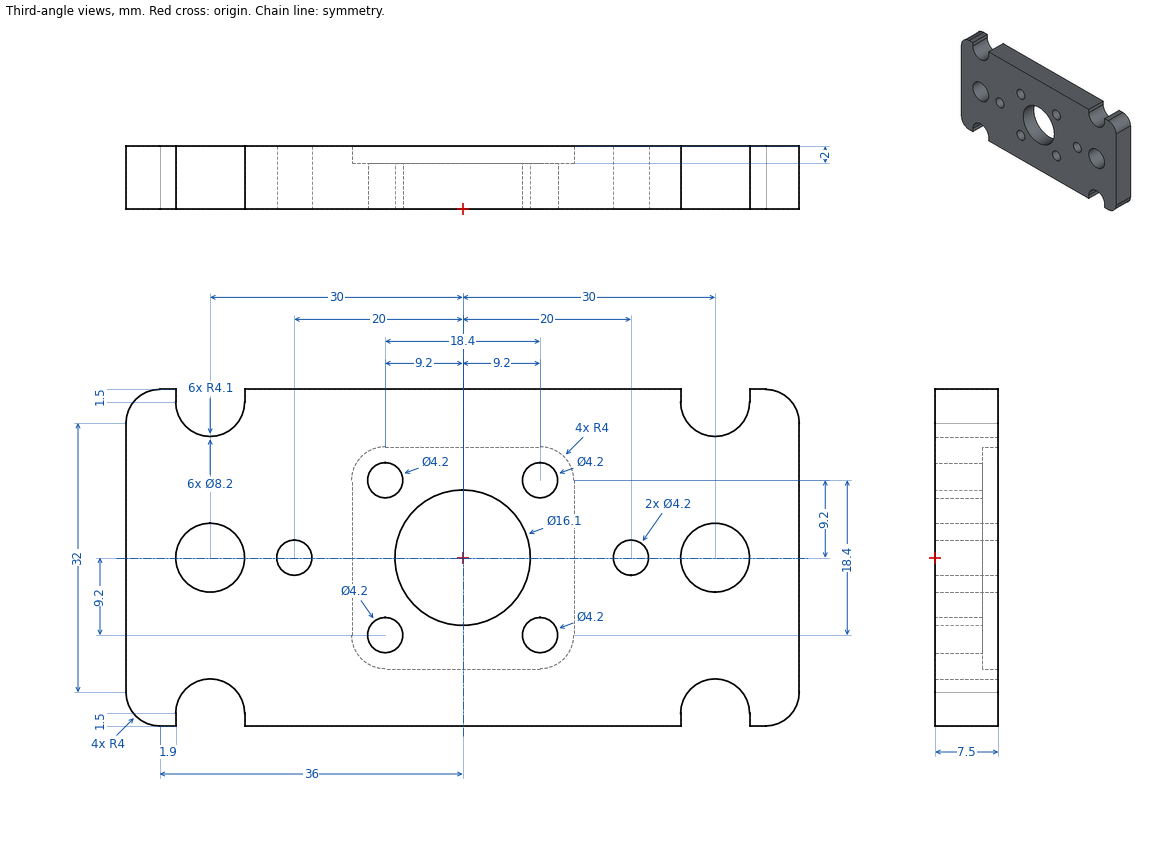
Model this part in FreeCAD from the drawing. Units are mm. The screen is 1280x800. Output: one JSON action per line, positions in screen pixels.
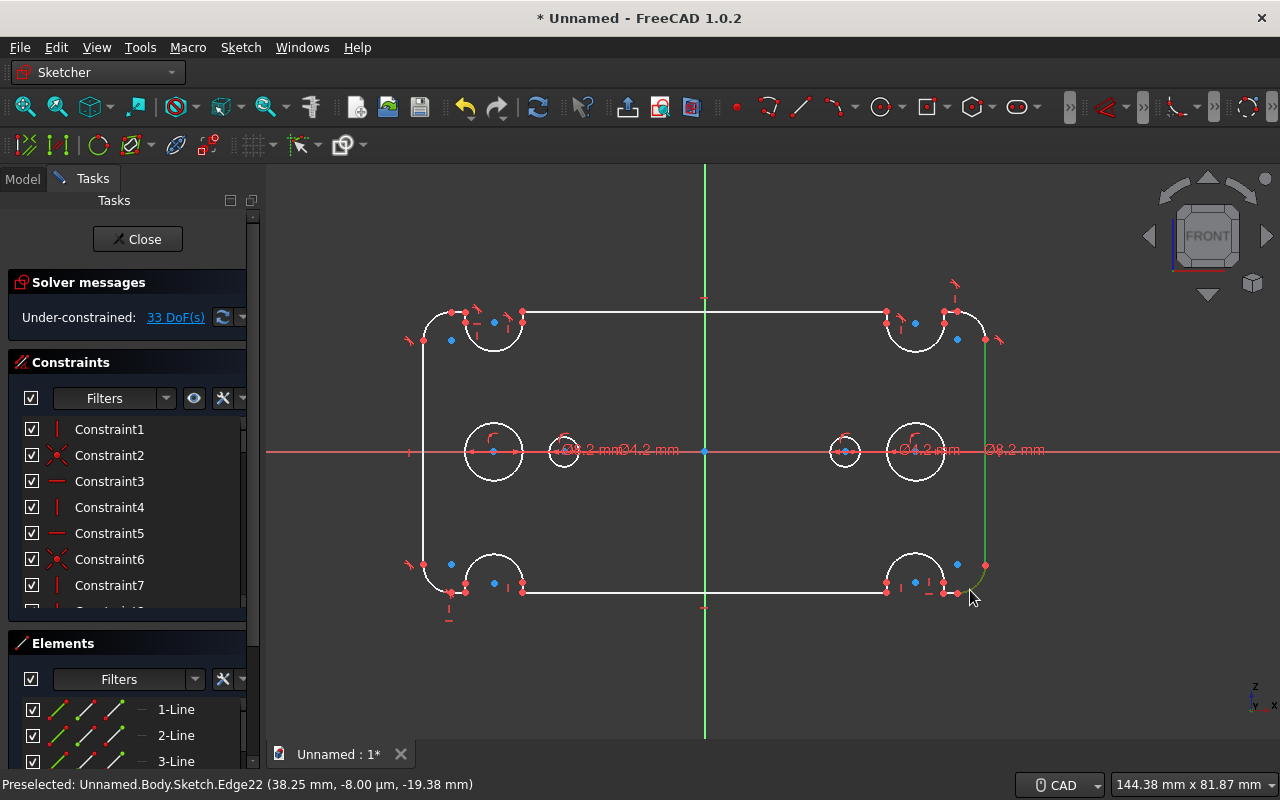
{"action": "key", "text": "t"}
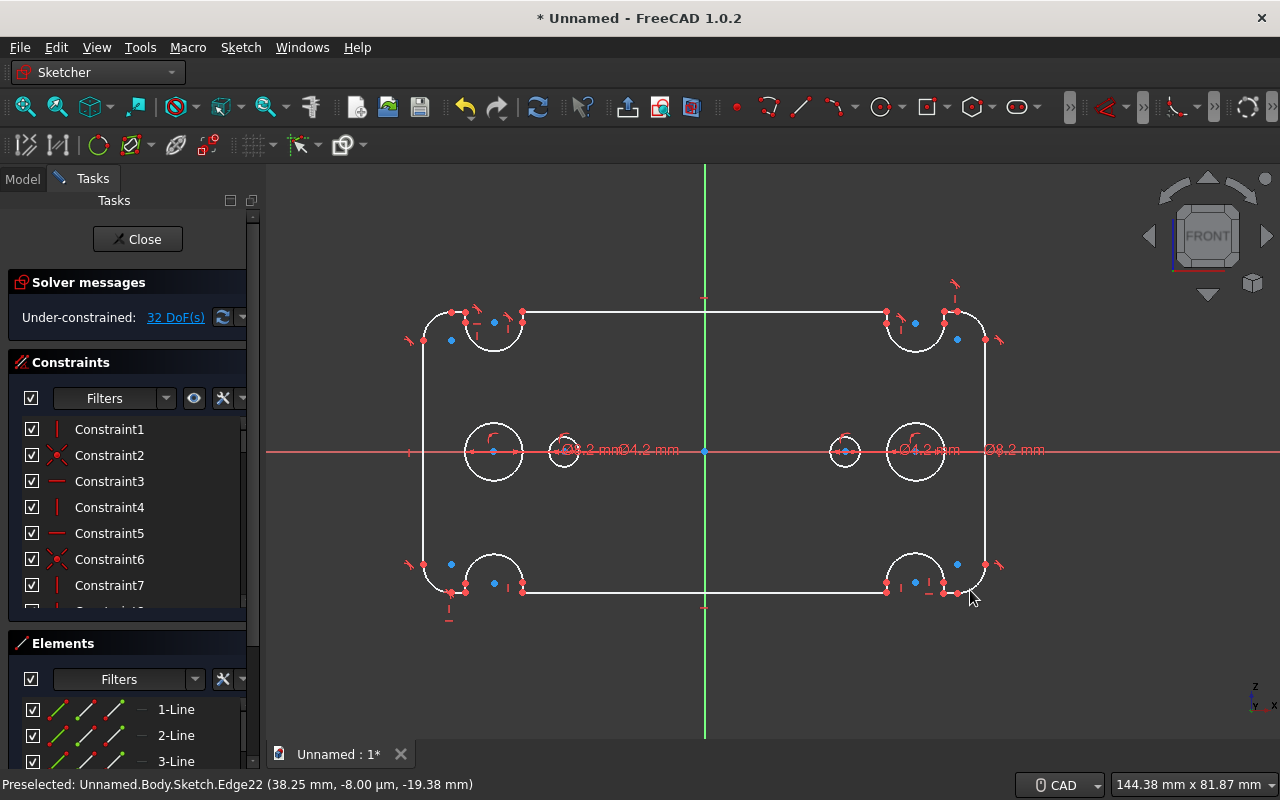
{"action": "scroll", "coordinate": [951, 593], "scroll_direction": "up", "scroll_amount": 4}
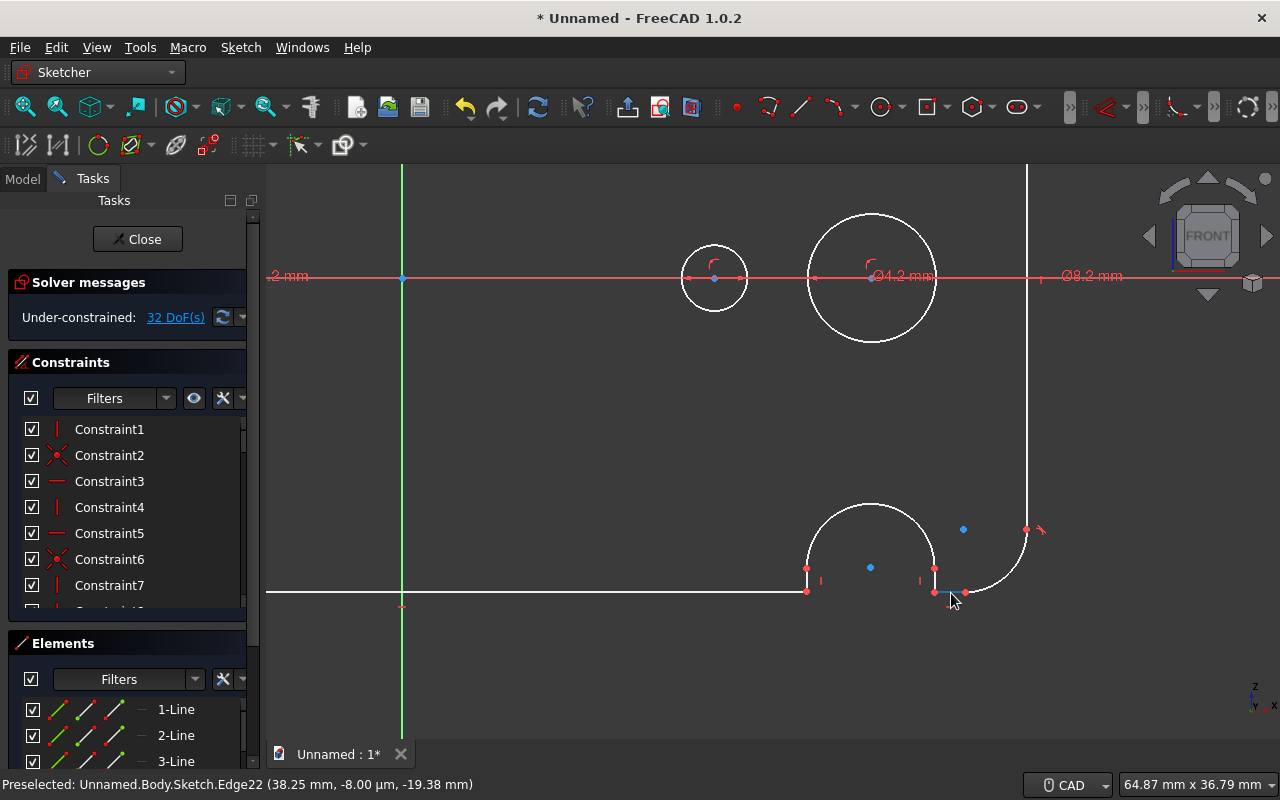
{"action": "left_click", "coordinate": [950, 592]}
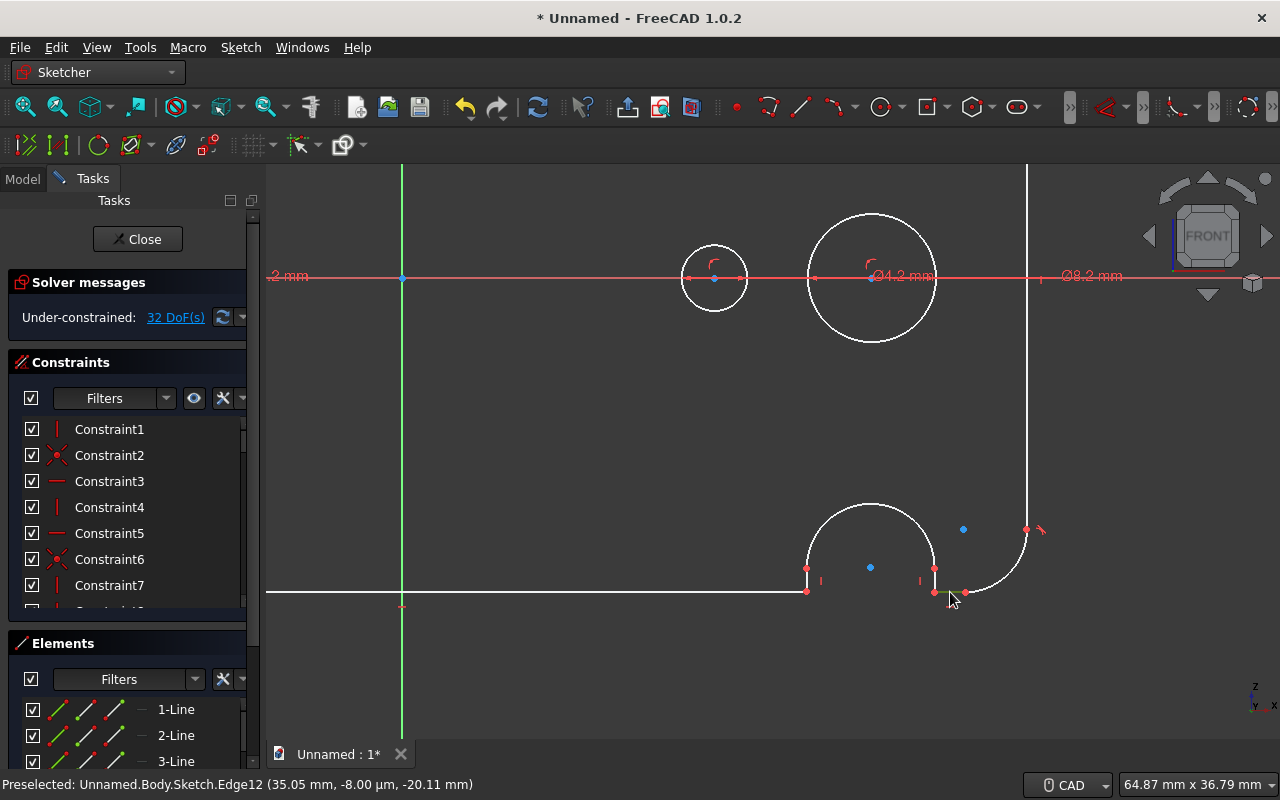
{"action": "left_click", "coordinate": [994, 585]}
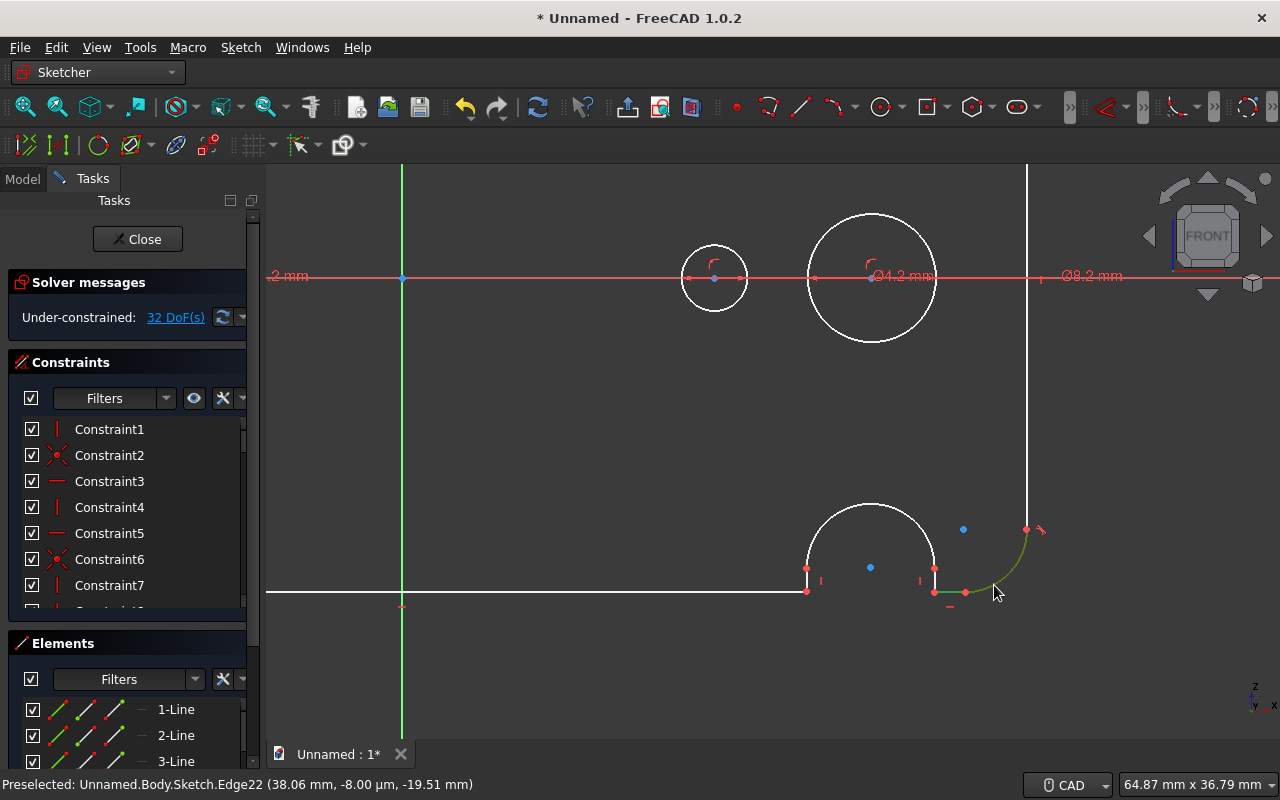
{"action": "key", "text": "t"}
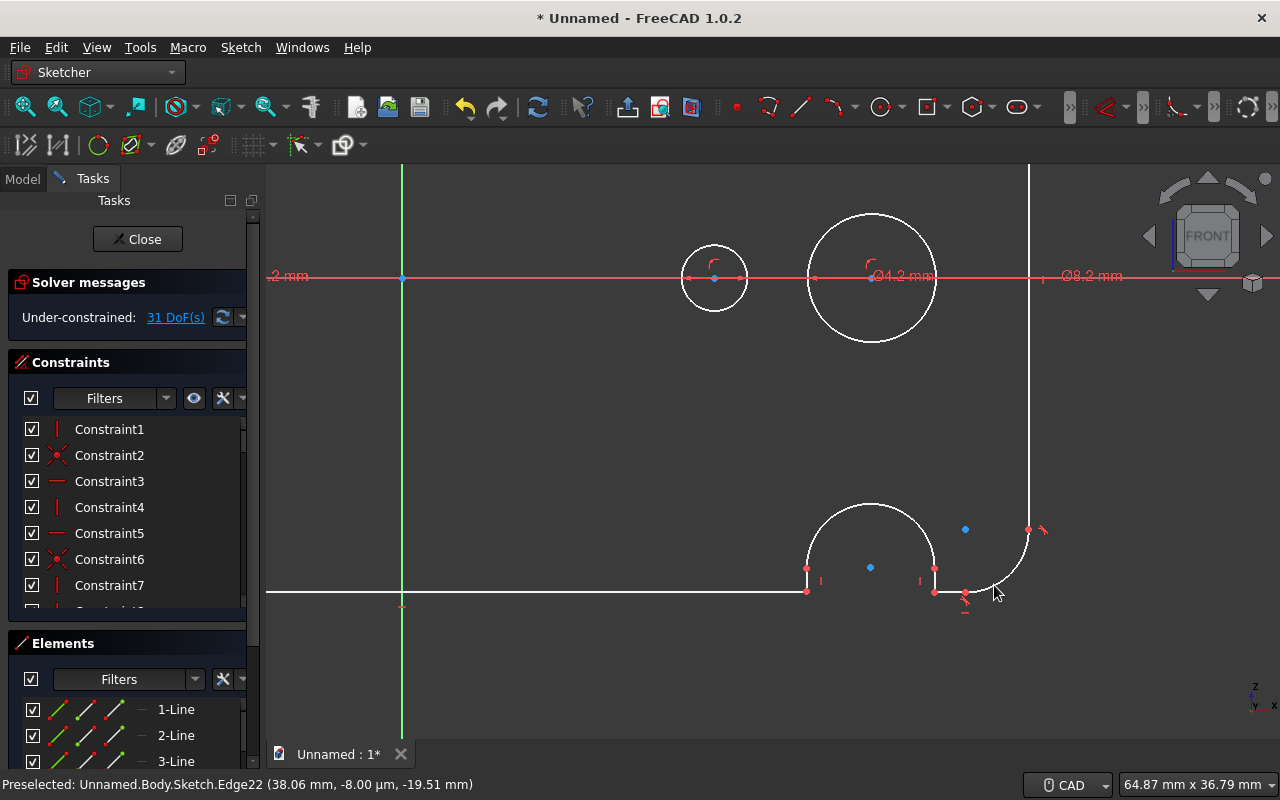
{"action": "scroll", "coordinate": [935, 583], "scroll_direction": "up", "scroll_amount": 2}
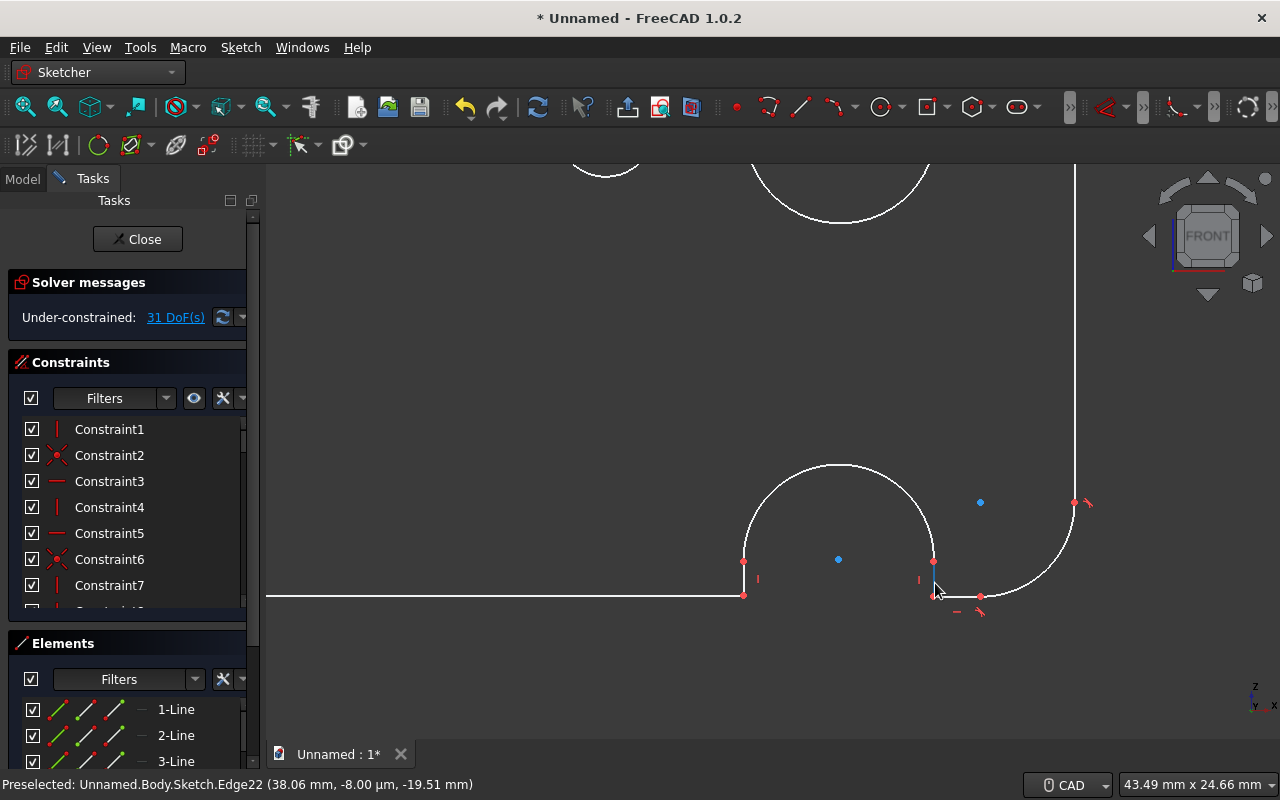
{"action": "left_click", "coordinate": [934, 583]}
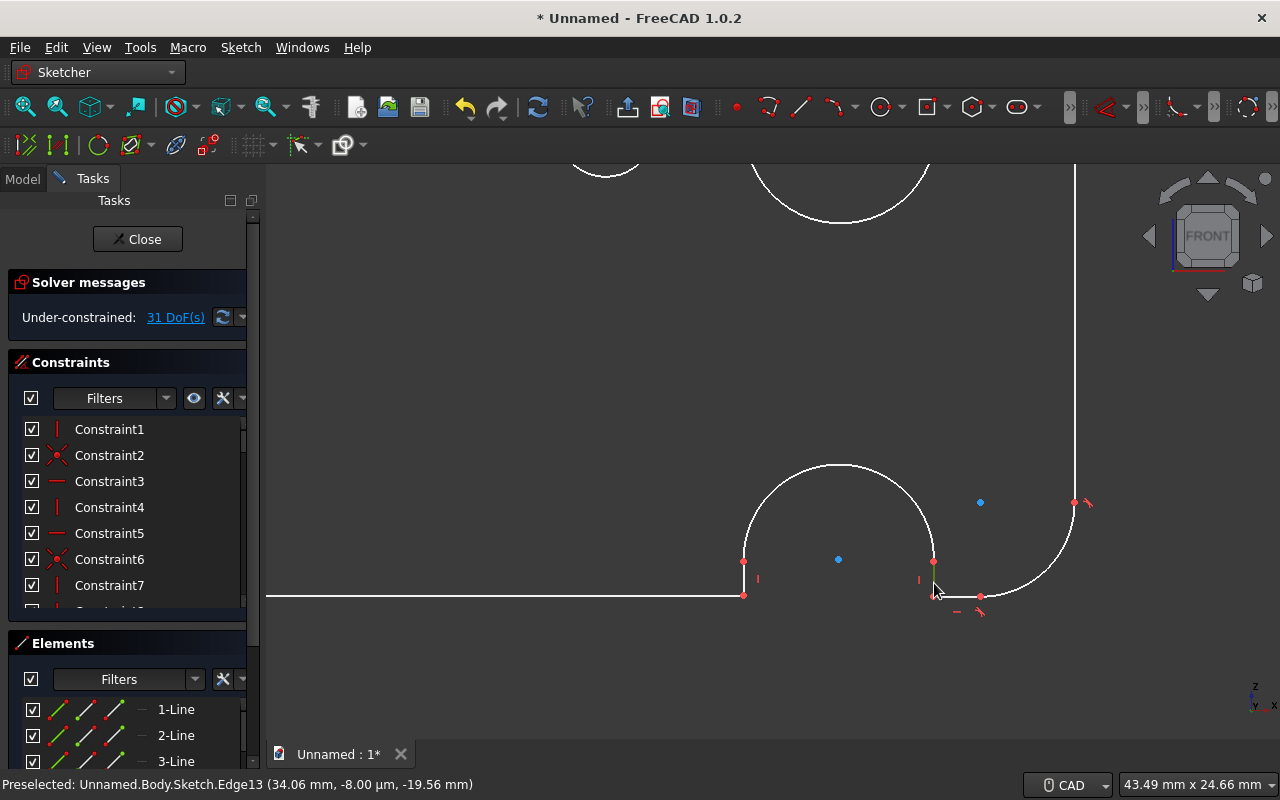
{"action": "scroll", "coordinate": [948, 591], "scroll_direction": "down", "scroll_amount": 6}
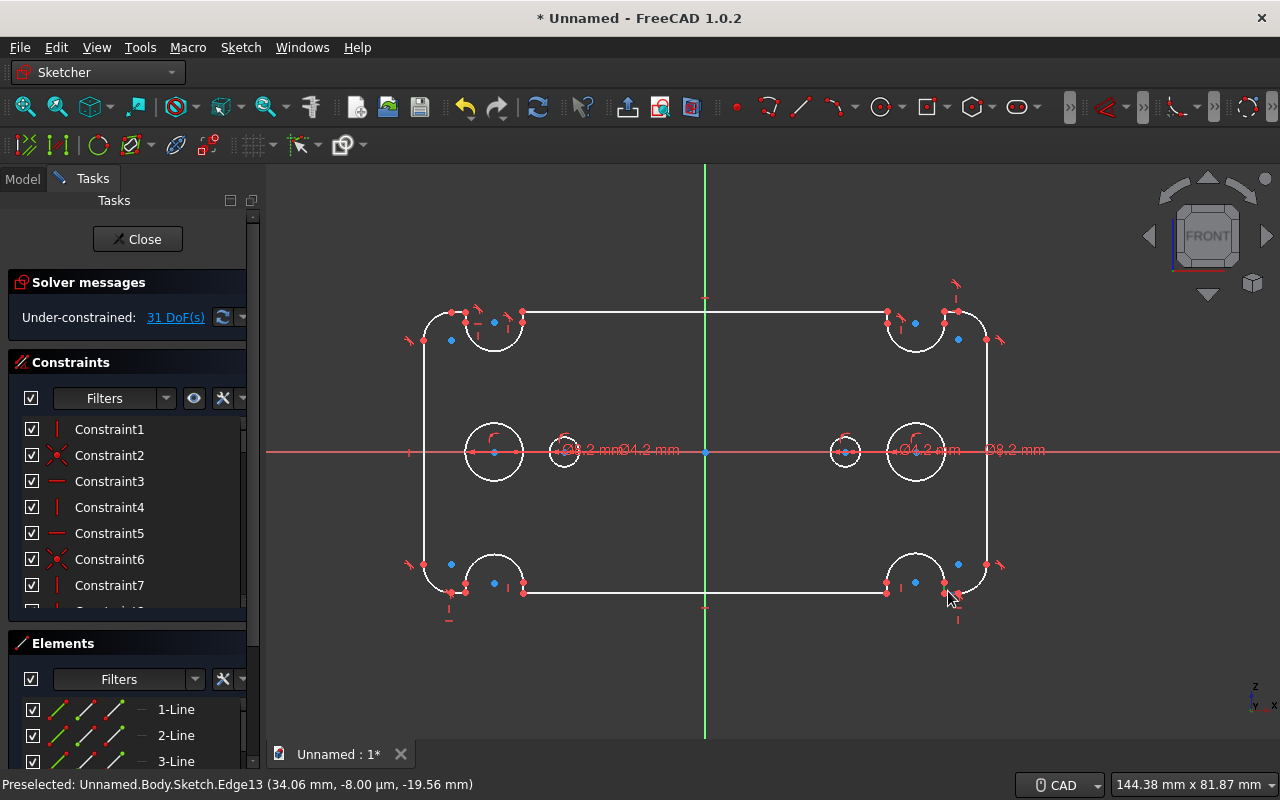
{"action": "left_click", "coordinate": [933, 559]}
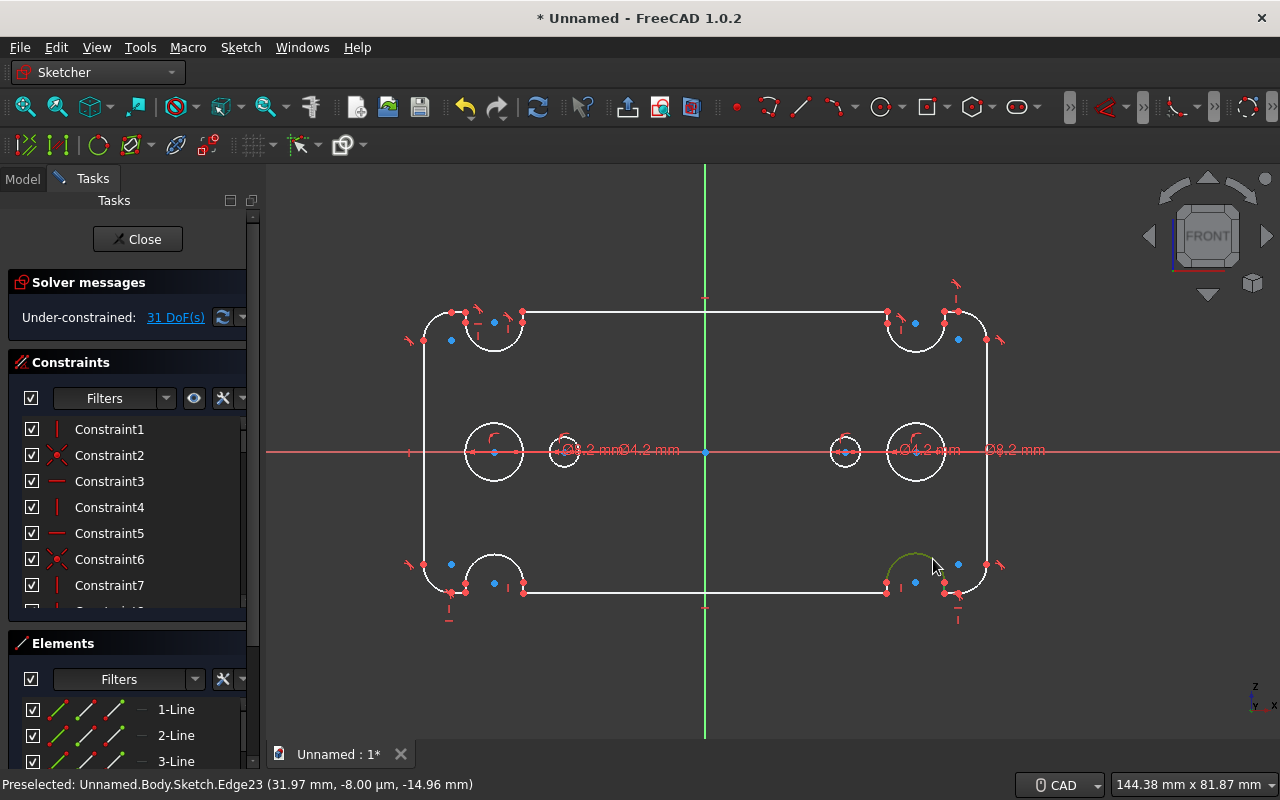
{"action": "key", "text": "t"}